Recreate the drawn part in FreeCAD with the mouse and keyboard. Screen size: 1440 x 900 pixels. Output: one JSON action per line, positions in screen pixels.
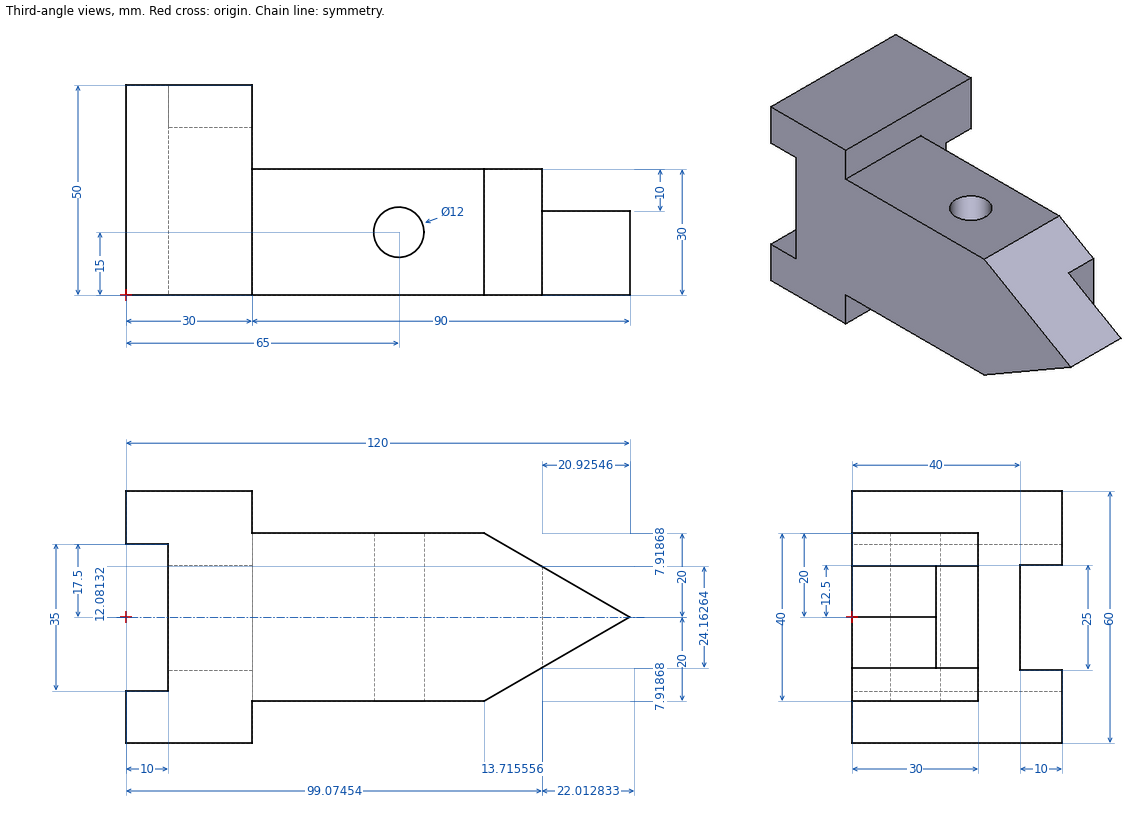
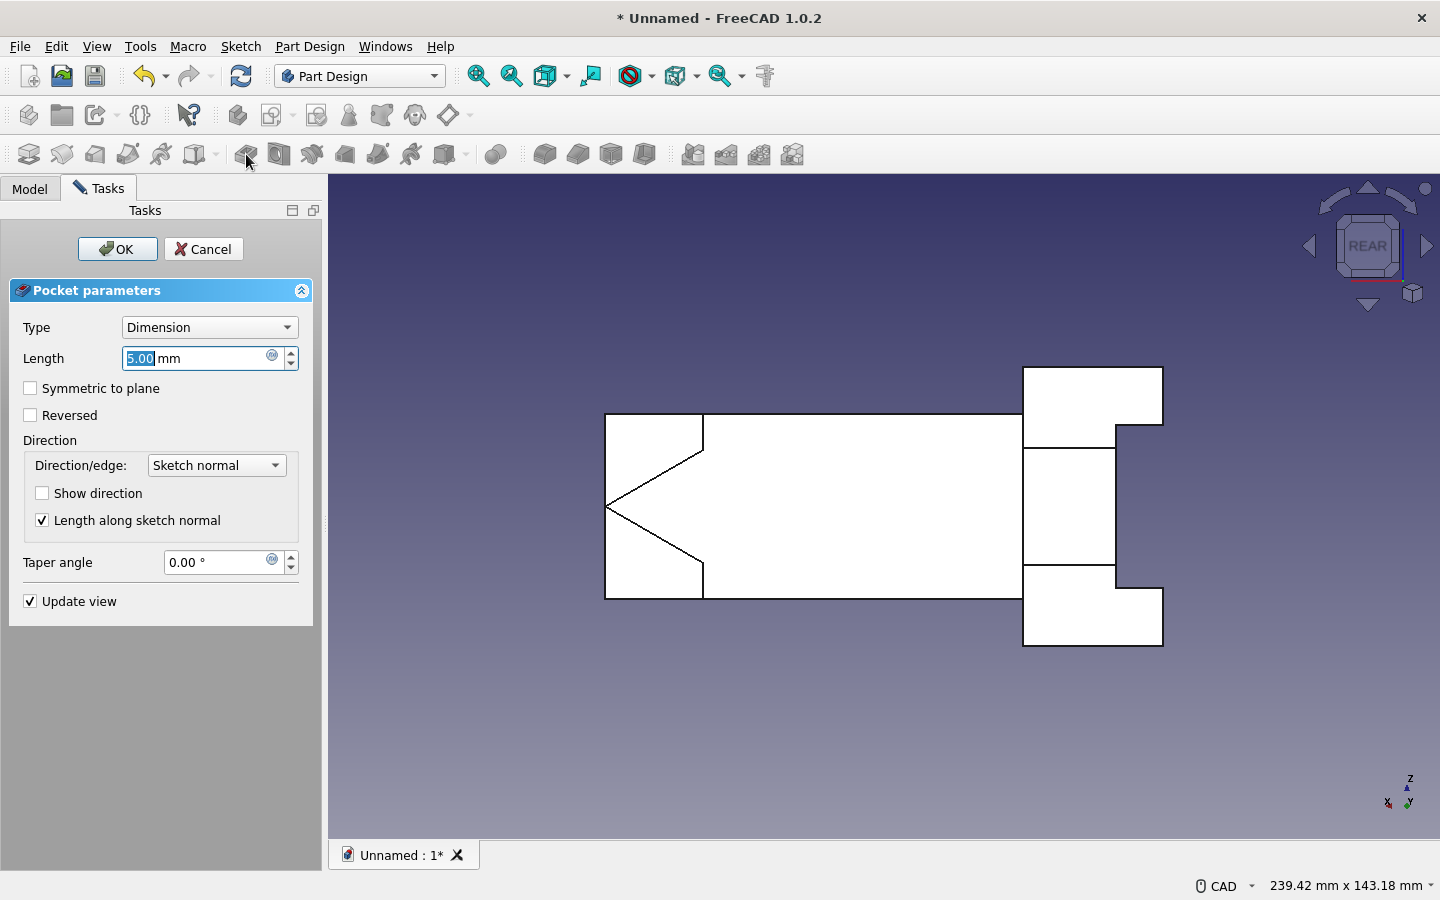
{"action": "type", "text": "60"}
{"action": "key", "text": "Tab"}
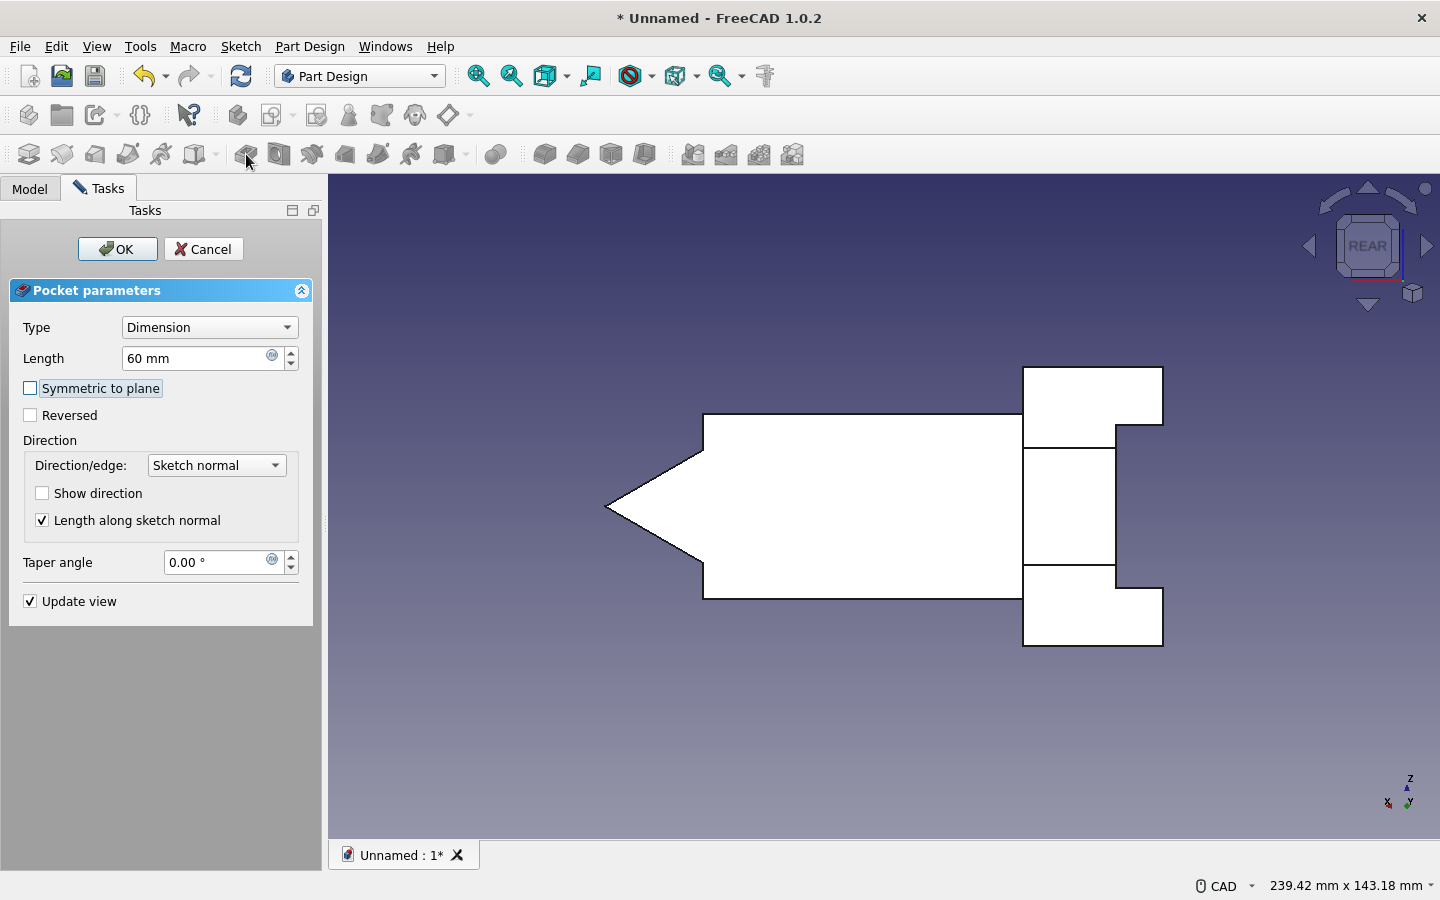
{"action": "left_click", "coordinate": [118, 249]}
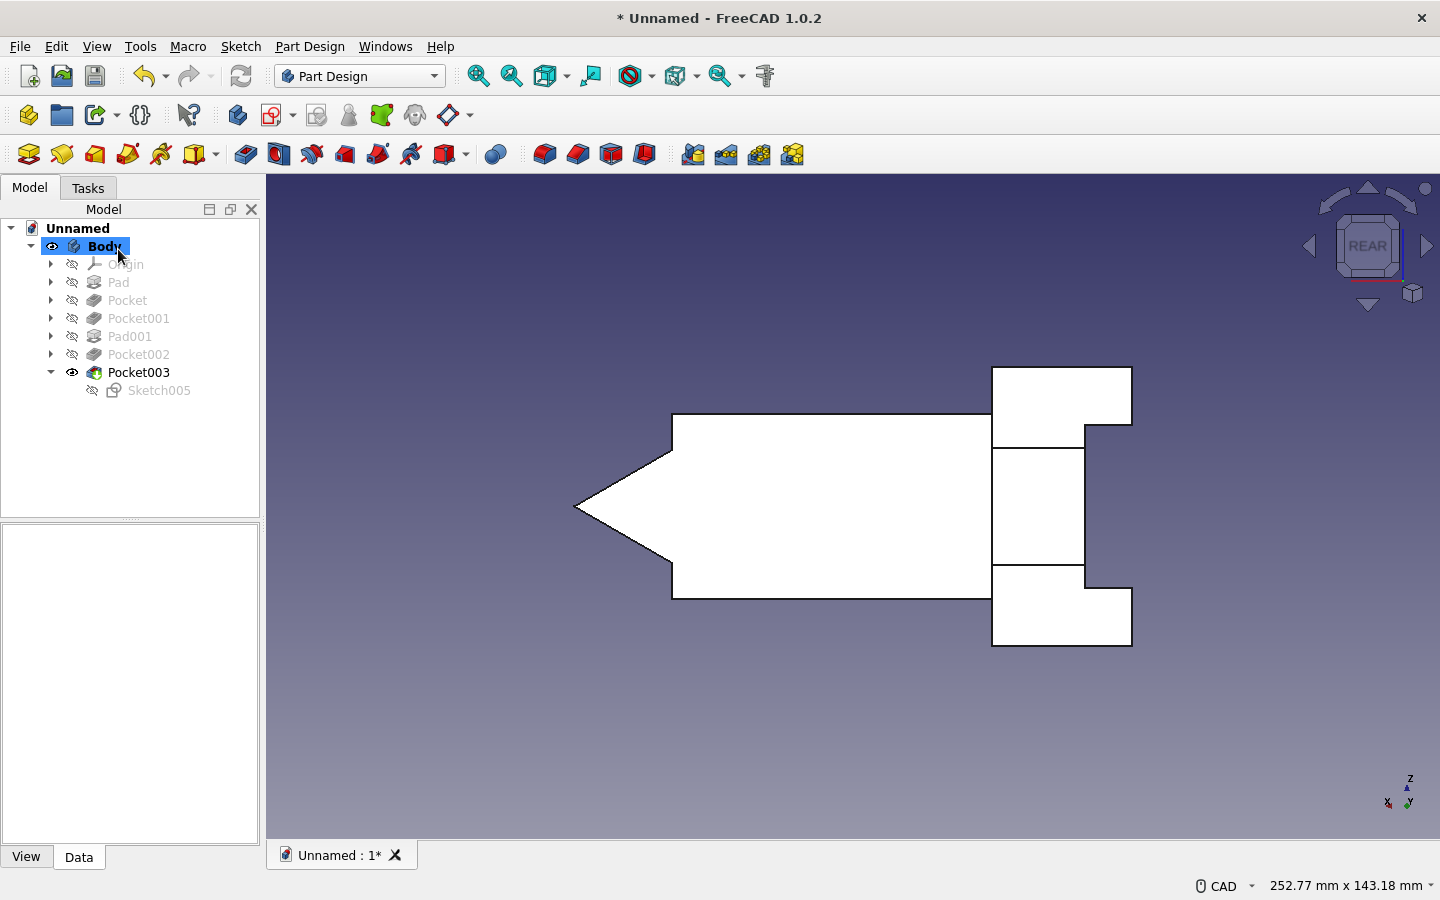
{"action": "left_click", "coordinate": [783, 506]}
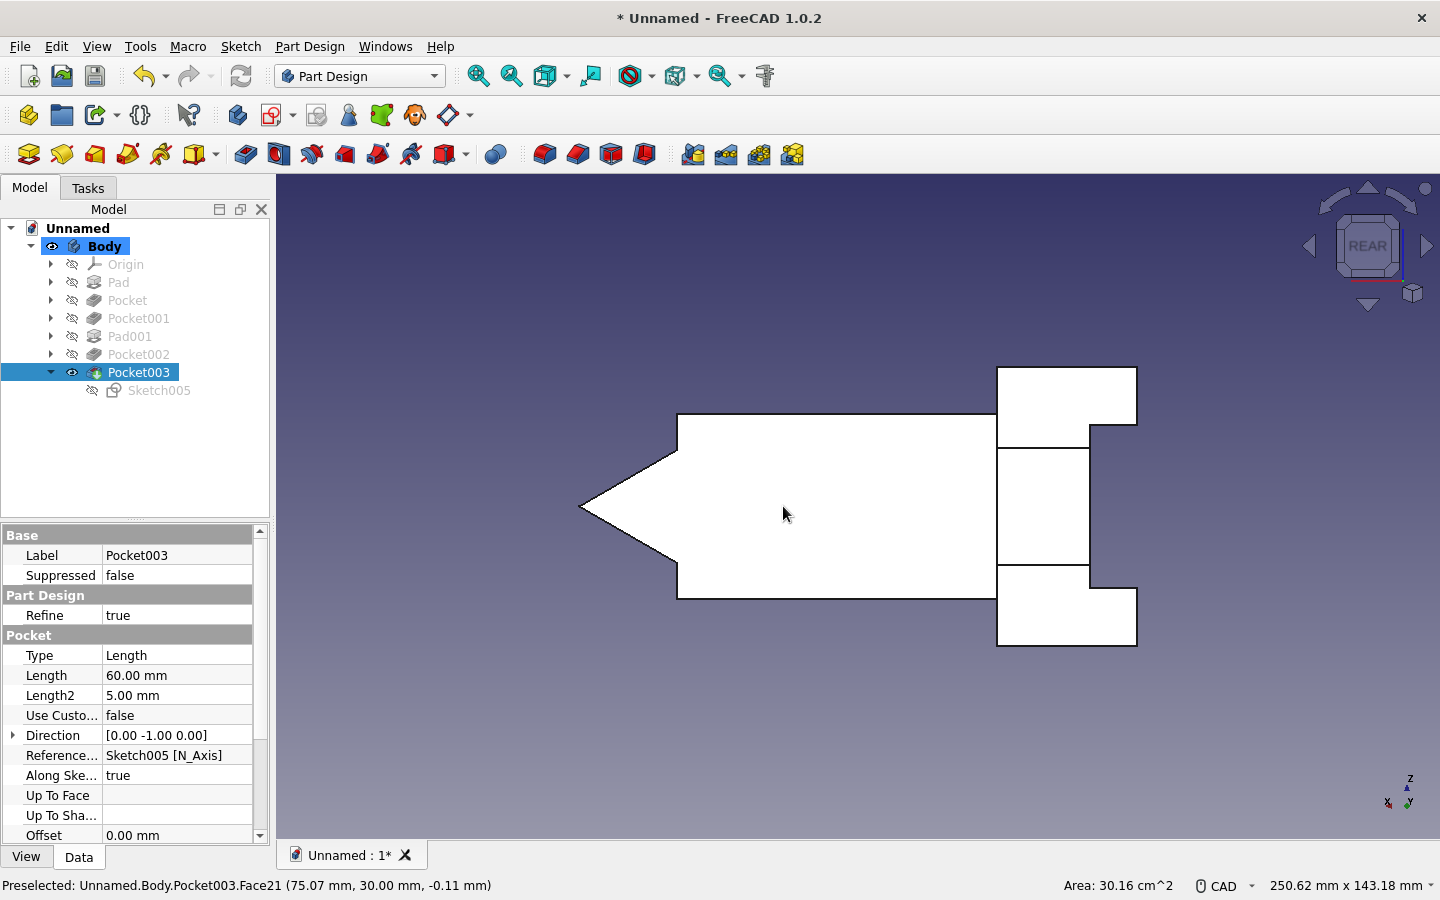
{"action": "left_click", "coordinate": [270, 116]}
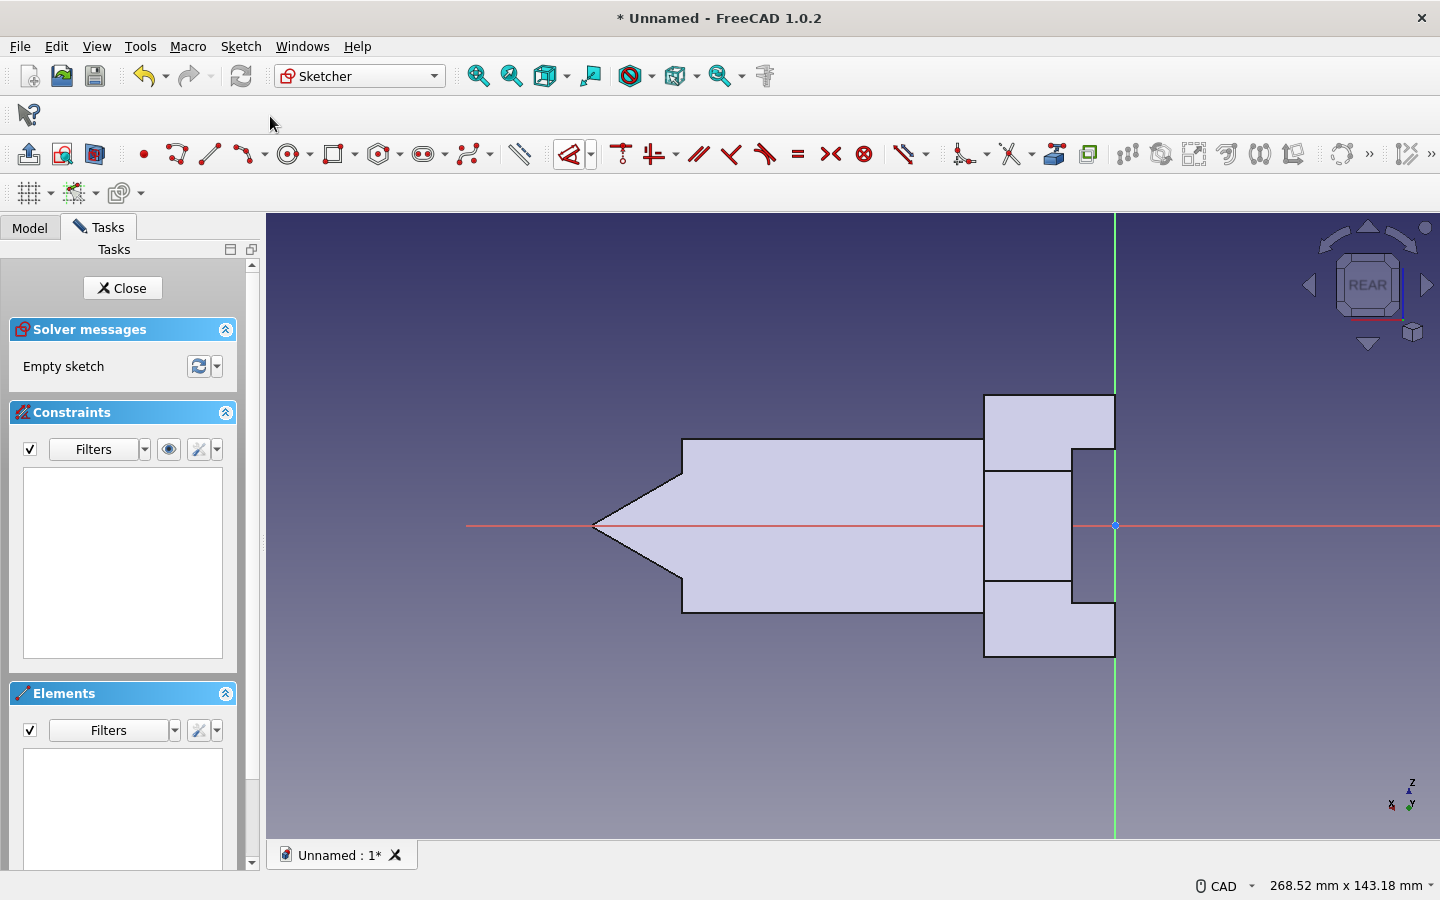
{"action": "scroll", "coordinate": [585, 526], "scroll_direction": "up", "scroll_amount": 7}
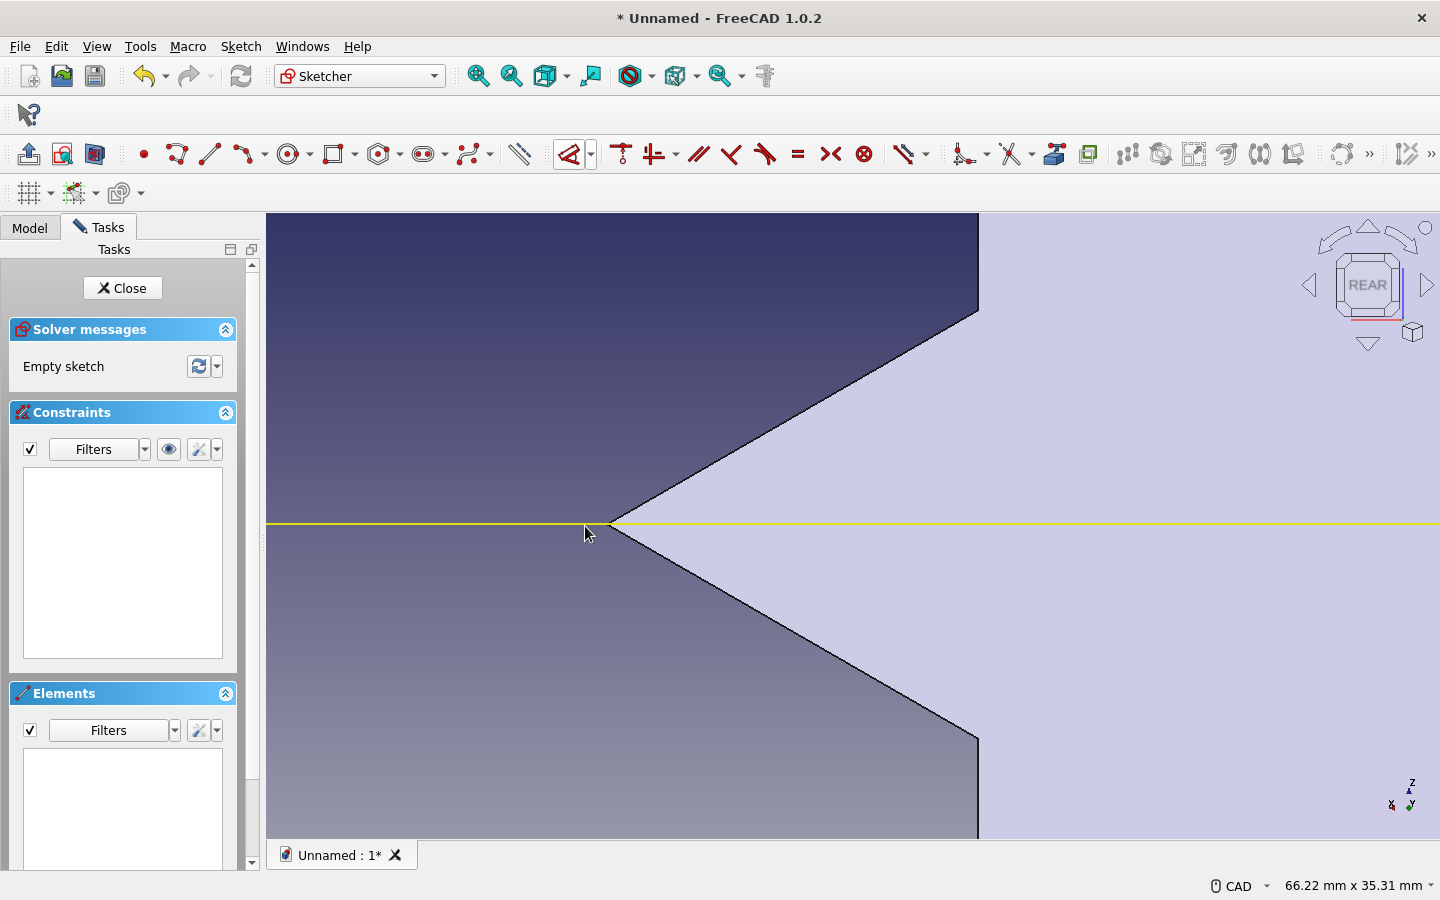
{"action": "left_click", "coordinate": [332, 154]}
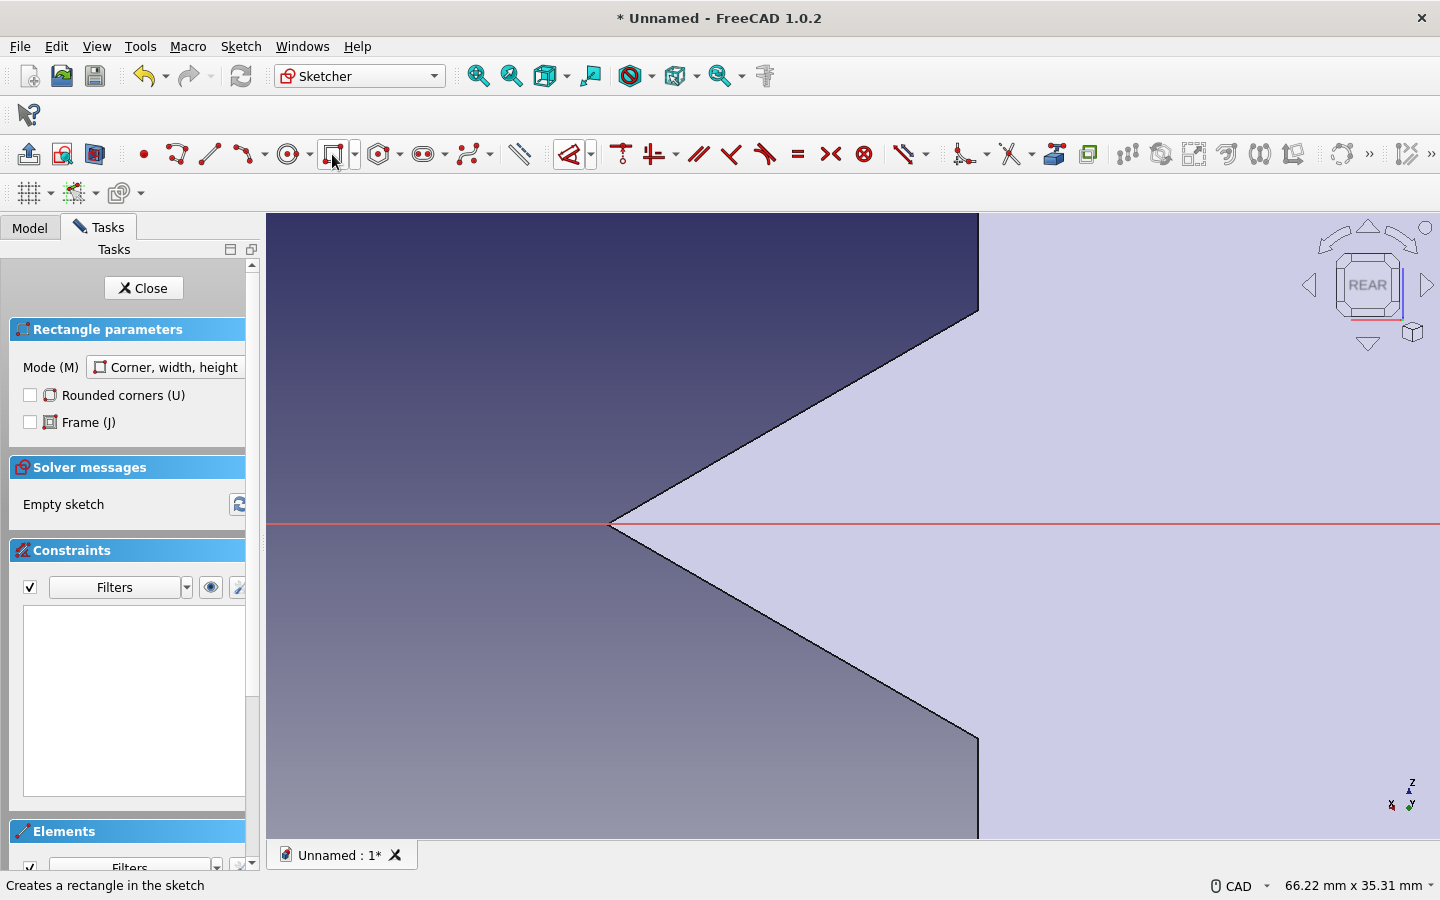
{"action": "left_click", "coordinate": [588, 310]}
{"action": "left_click", "coordinate": [978, 739]}
{"action": "key", "text": "Escape"}